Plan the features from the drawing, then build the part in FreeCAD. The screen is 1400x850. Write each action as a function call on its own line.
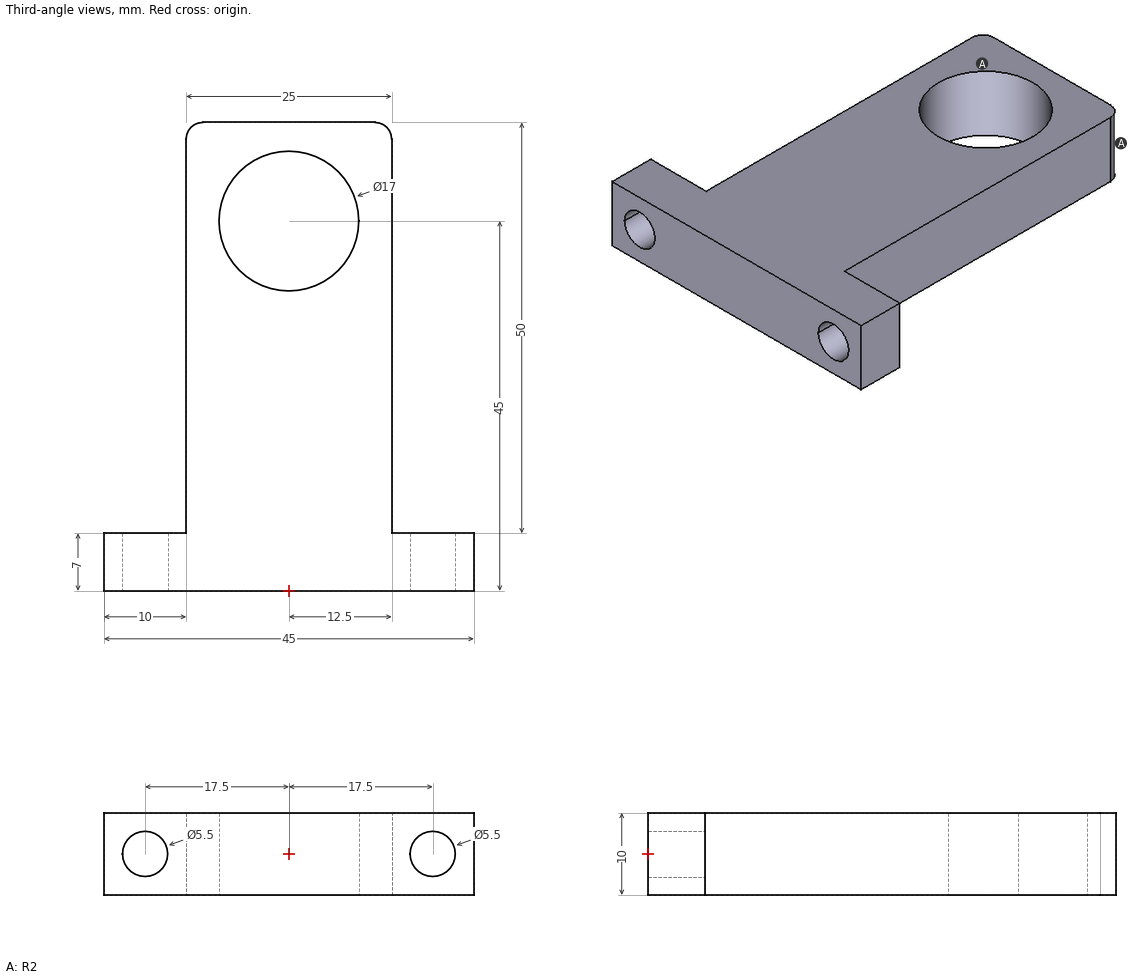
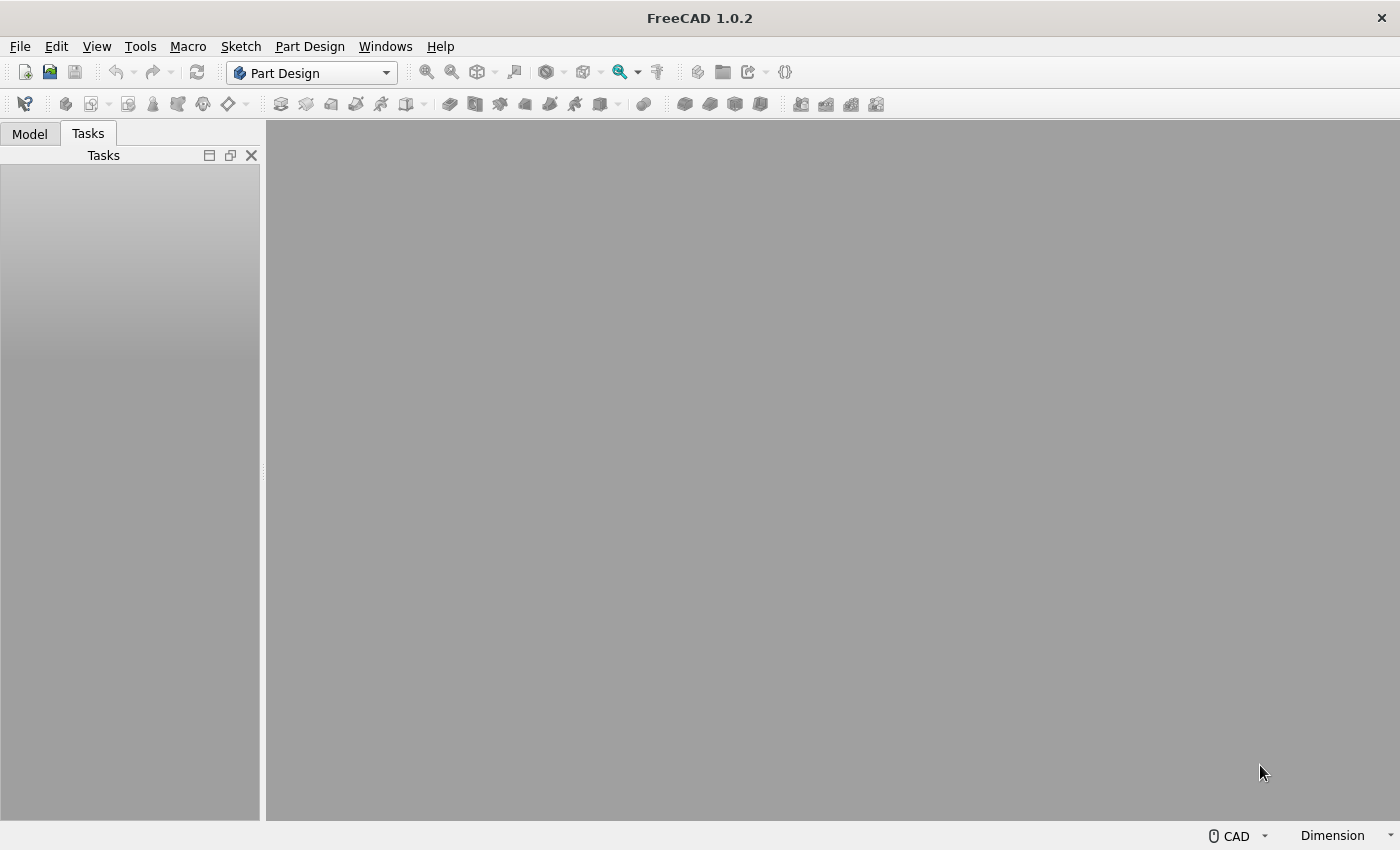
click(25, 72)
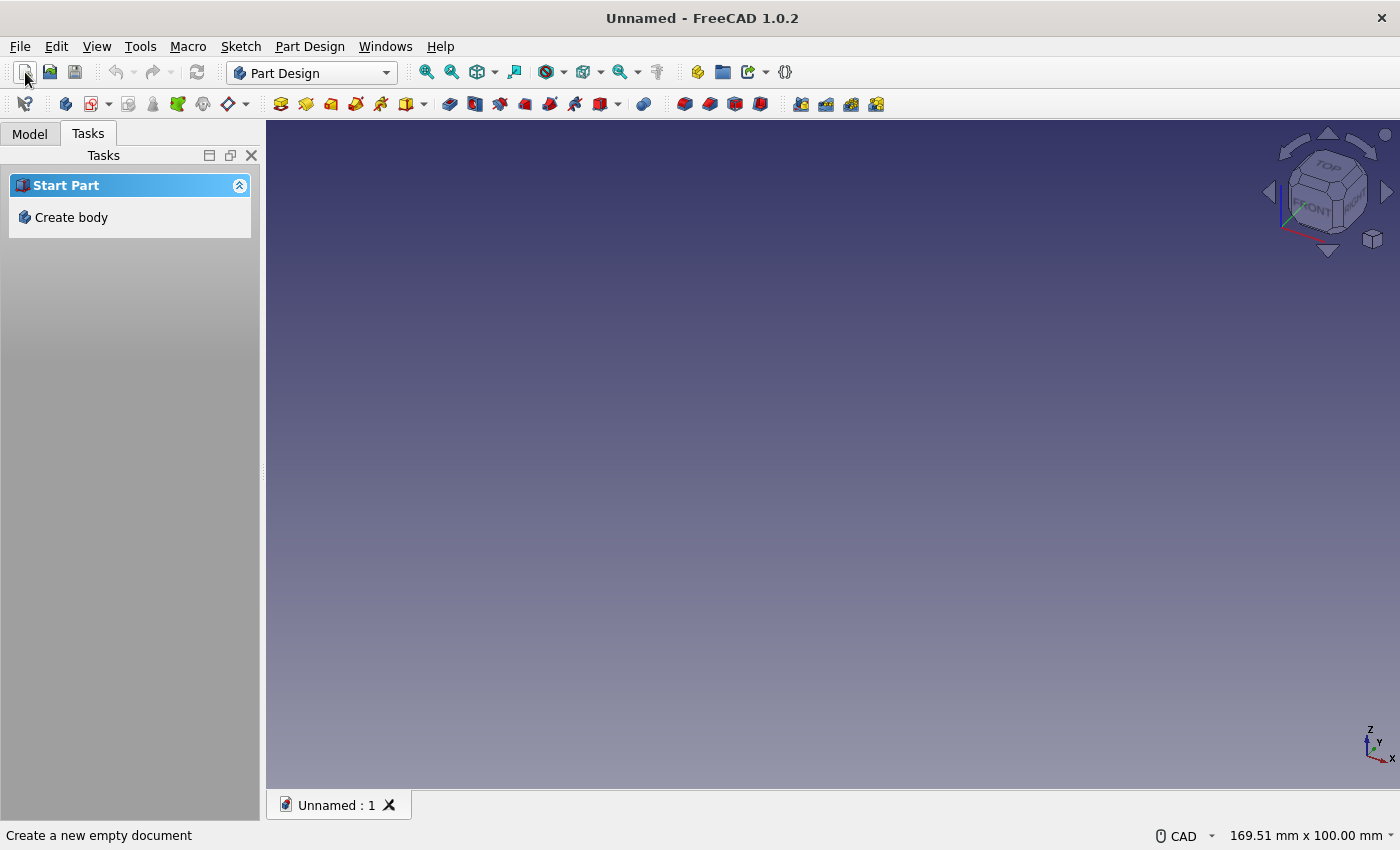
click(90, 104)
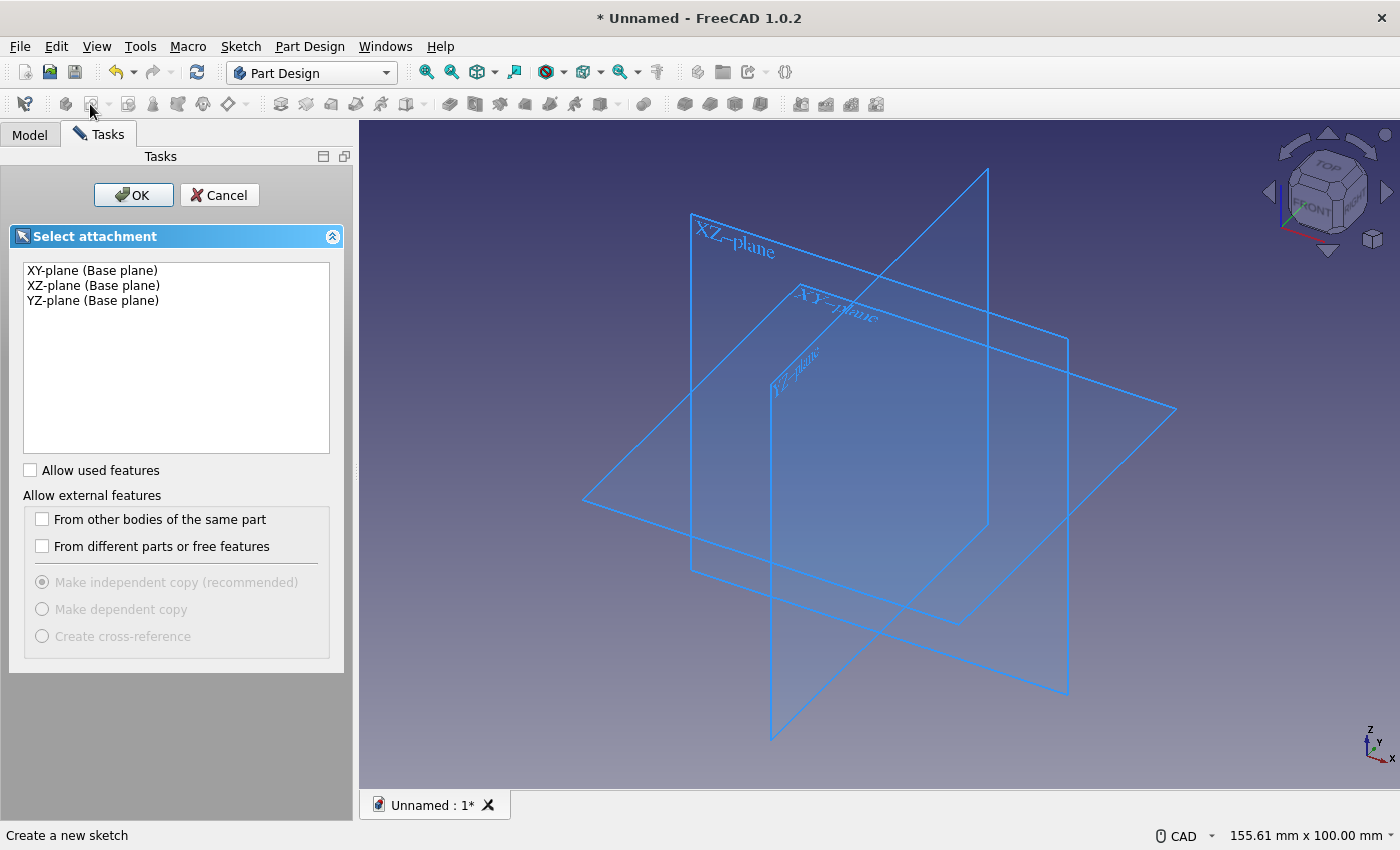
click(84, 270)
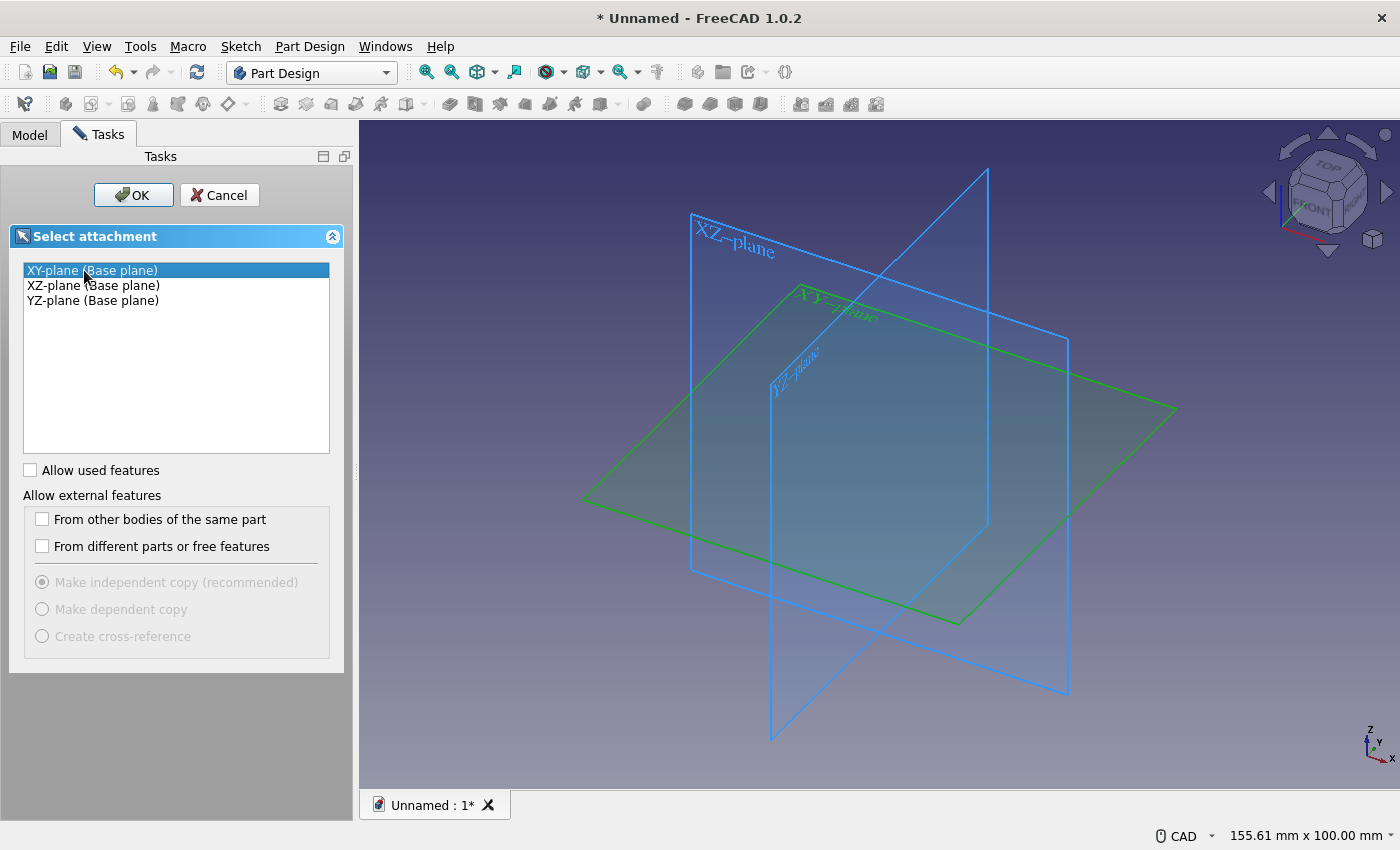
click(134, 195)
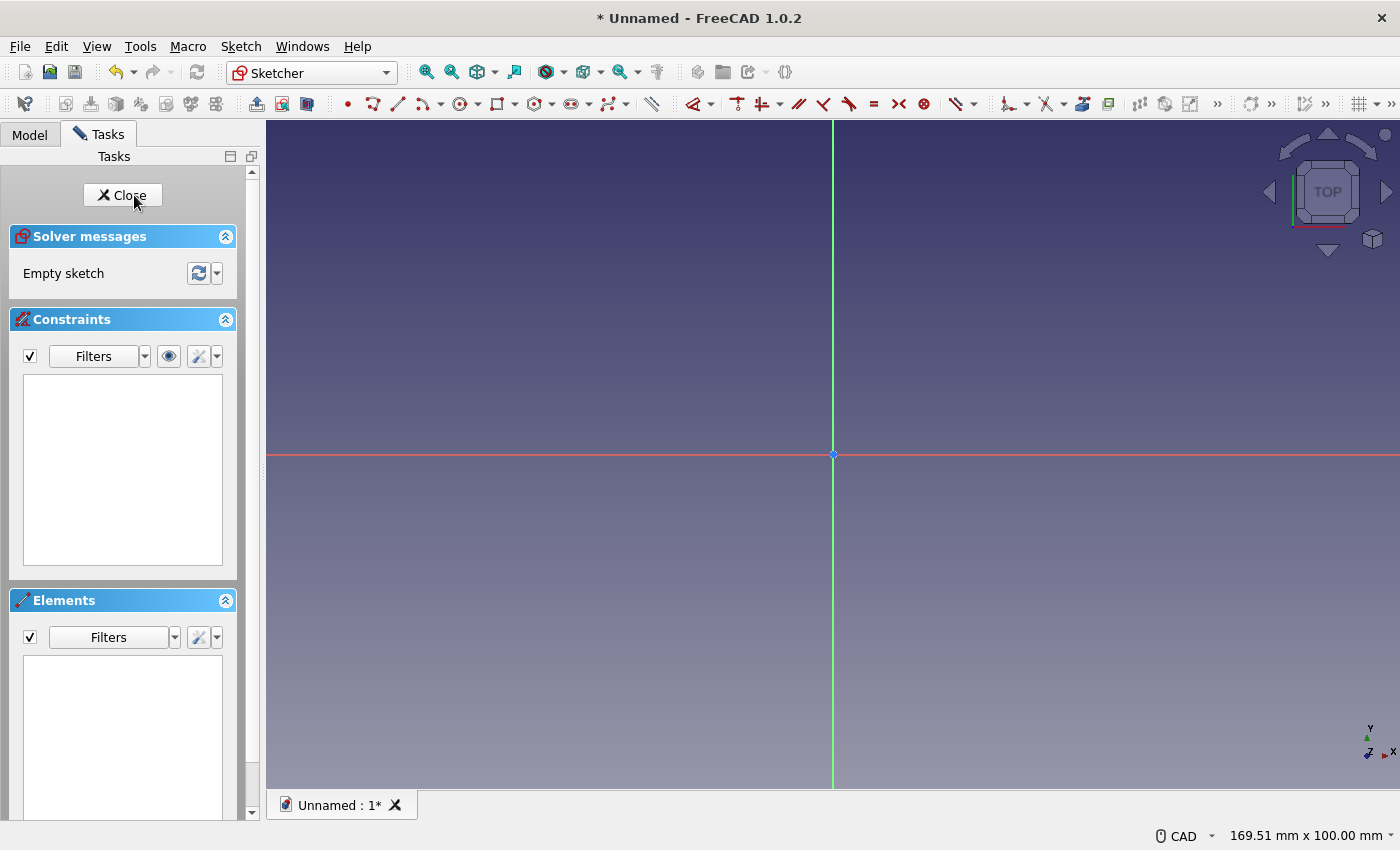
scroll(455, 761, down, 1)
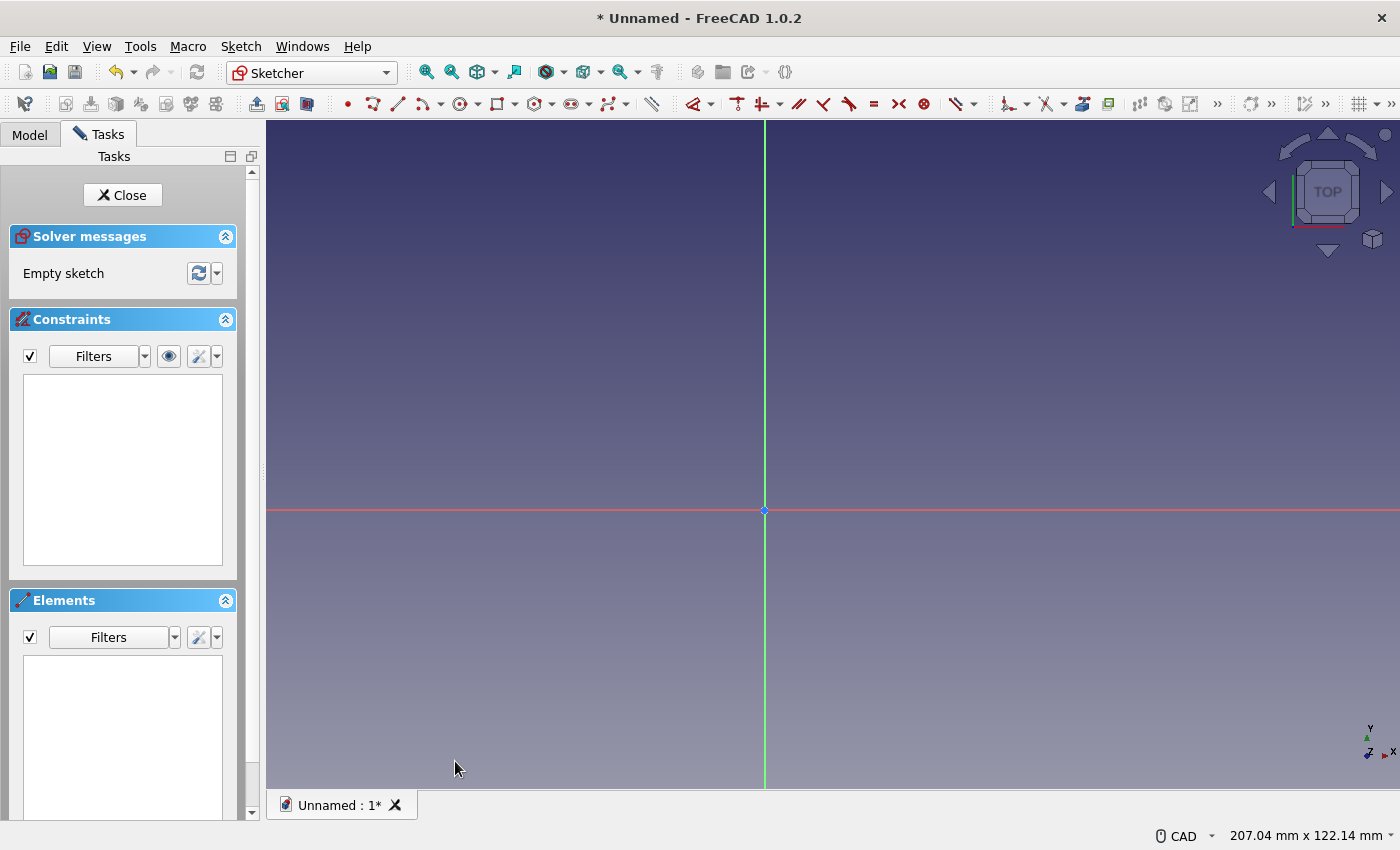
scroll(765, 150, up, 2)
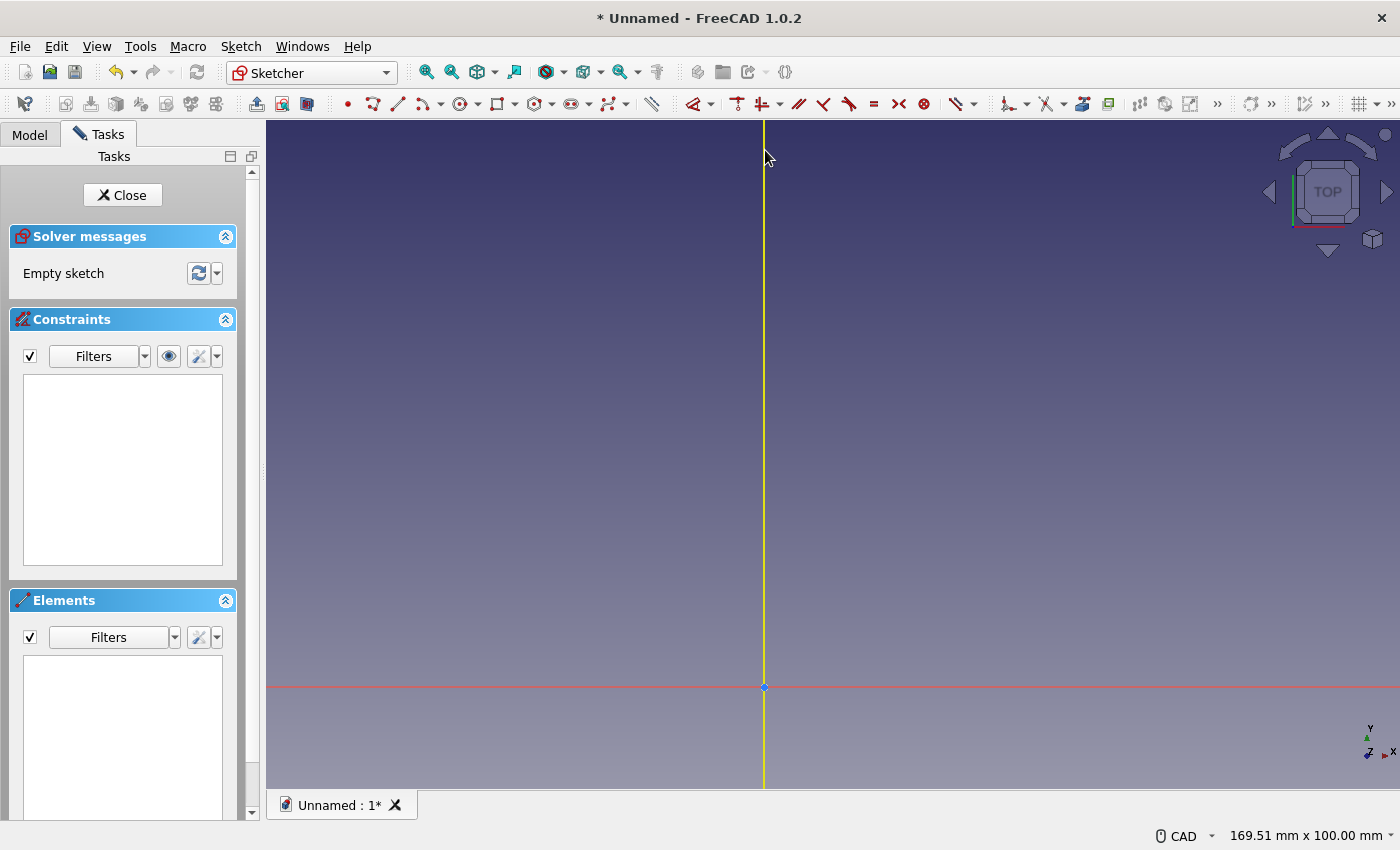
key(g)
key(m)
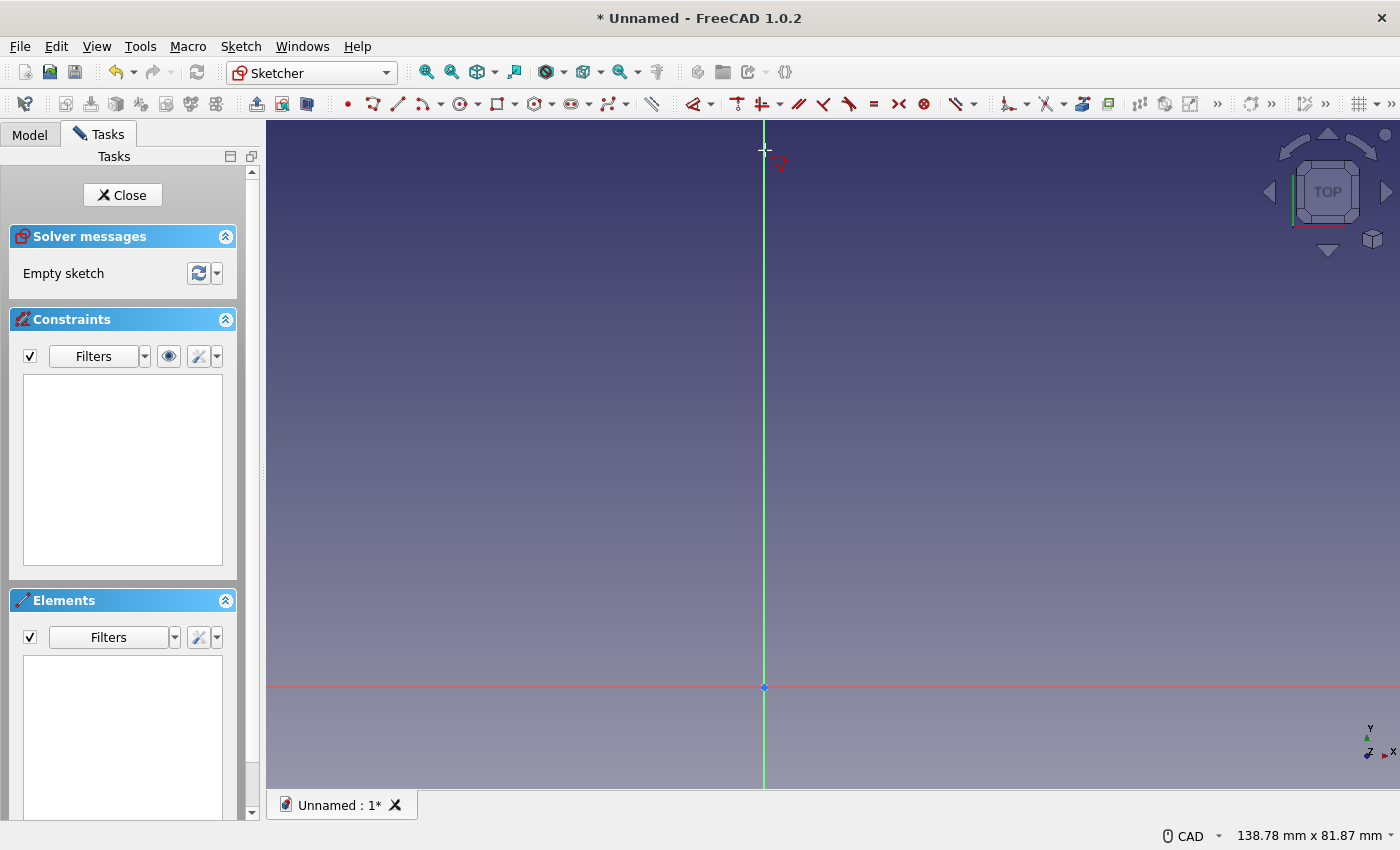
click(866, 630)
click(866, 222)
click(662, 222)
click(662, 630)
click(580, 630)
click(580, 687)
click(948, 678)
click(948, 630)
click(866, 631)